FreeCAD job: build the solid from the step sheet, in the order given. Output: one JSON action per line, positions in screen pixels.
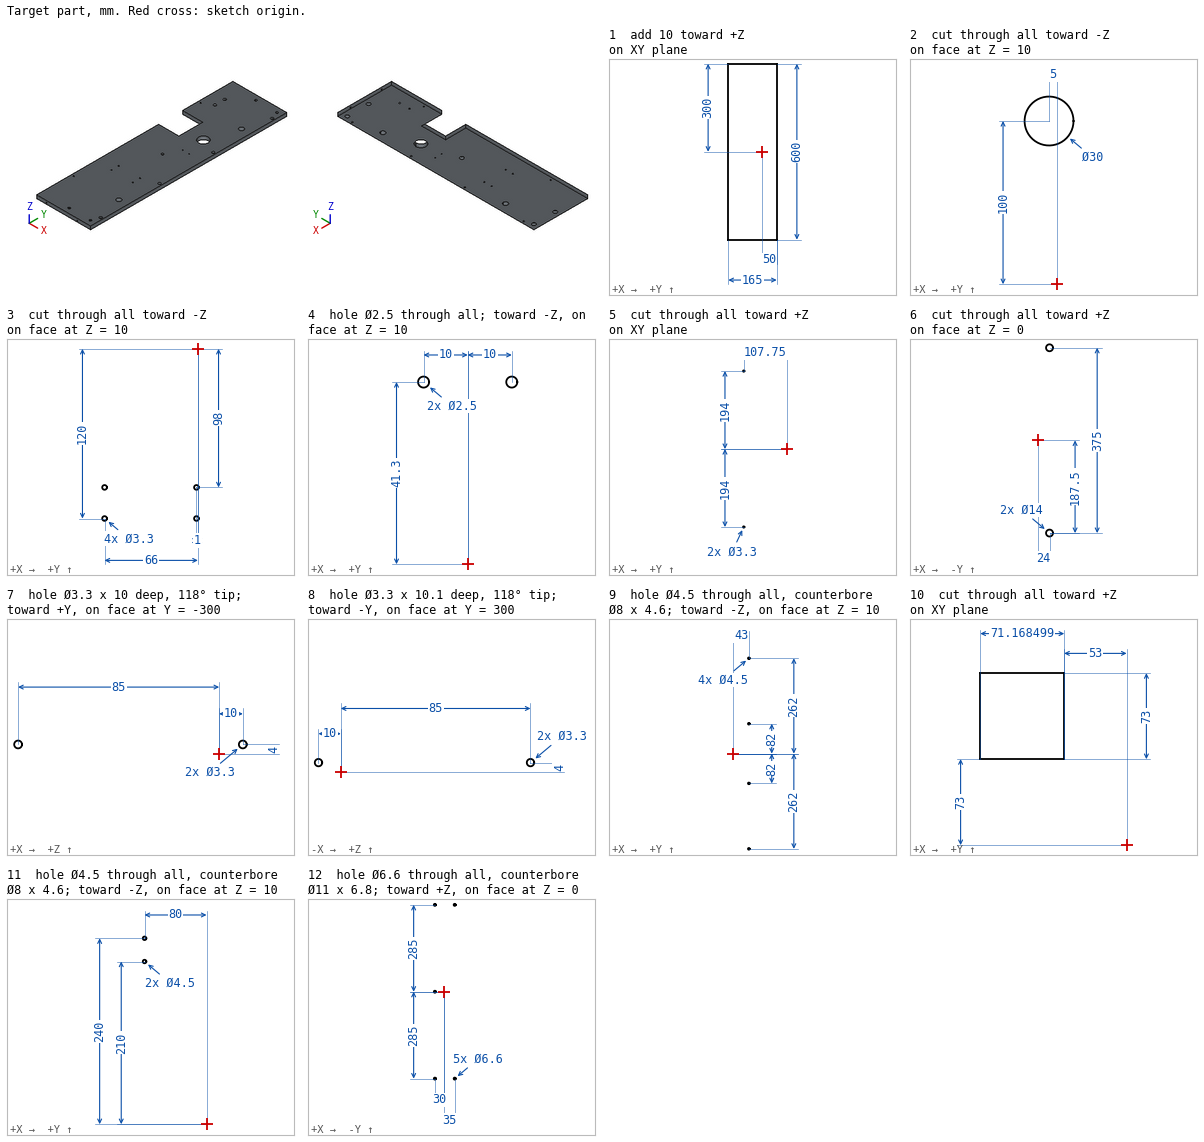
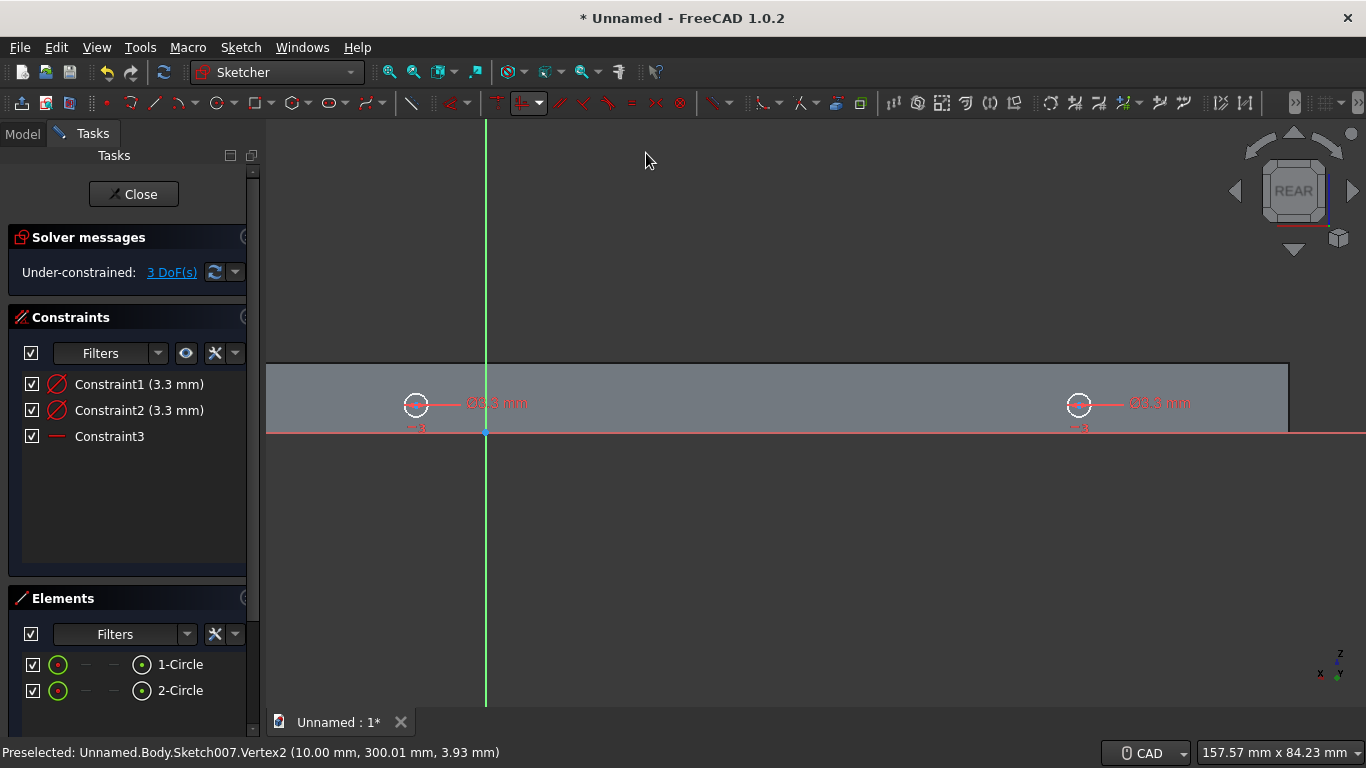
{"action": "left_click", "coordinate": [450, 104]}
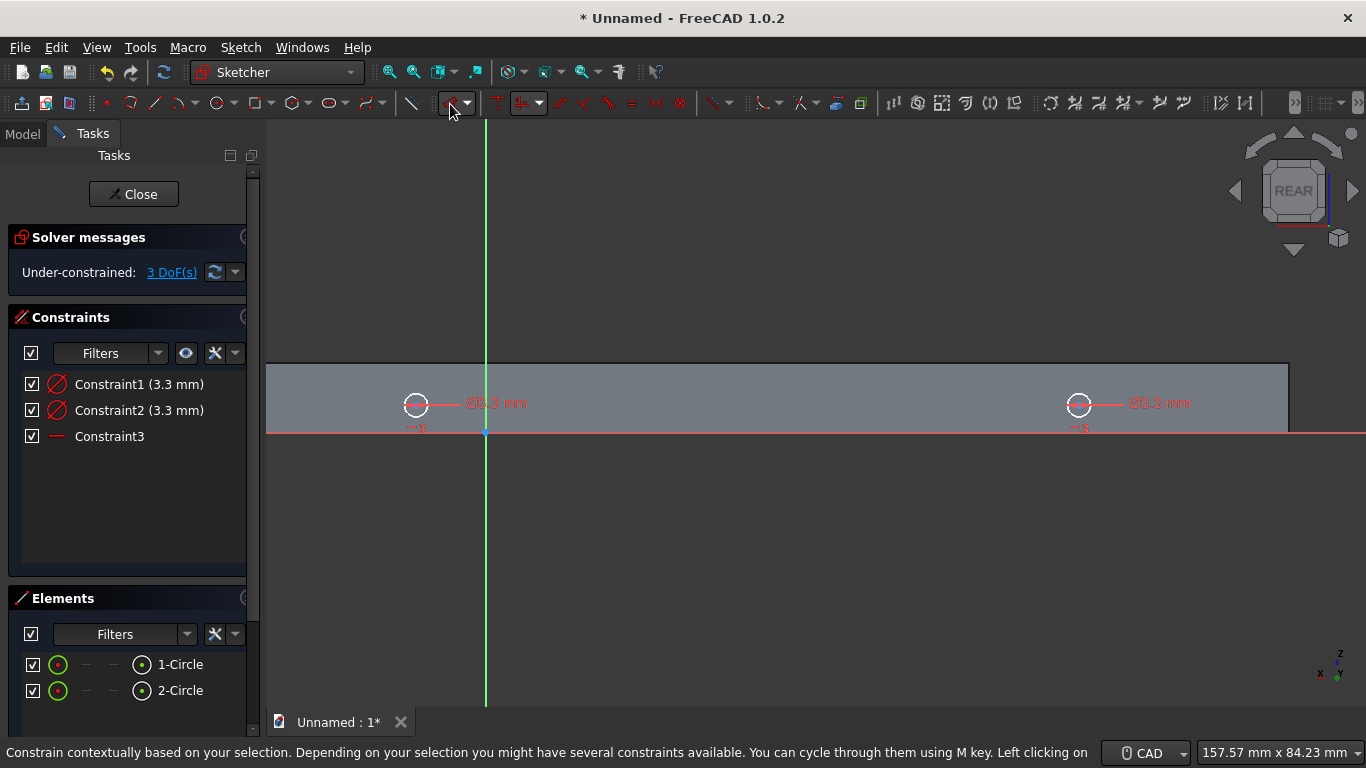
{"action": "scroll", "coordinate": [1079, 405], "scroll_direction": "up", "scroll_amount": 2}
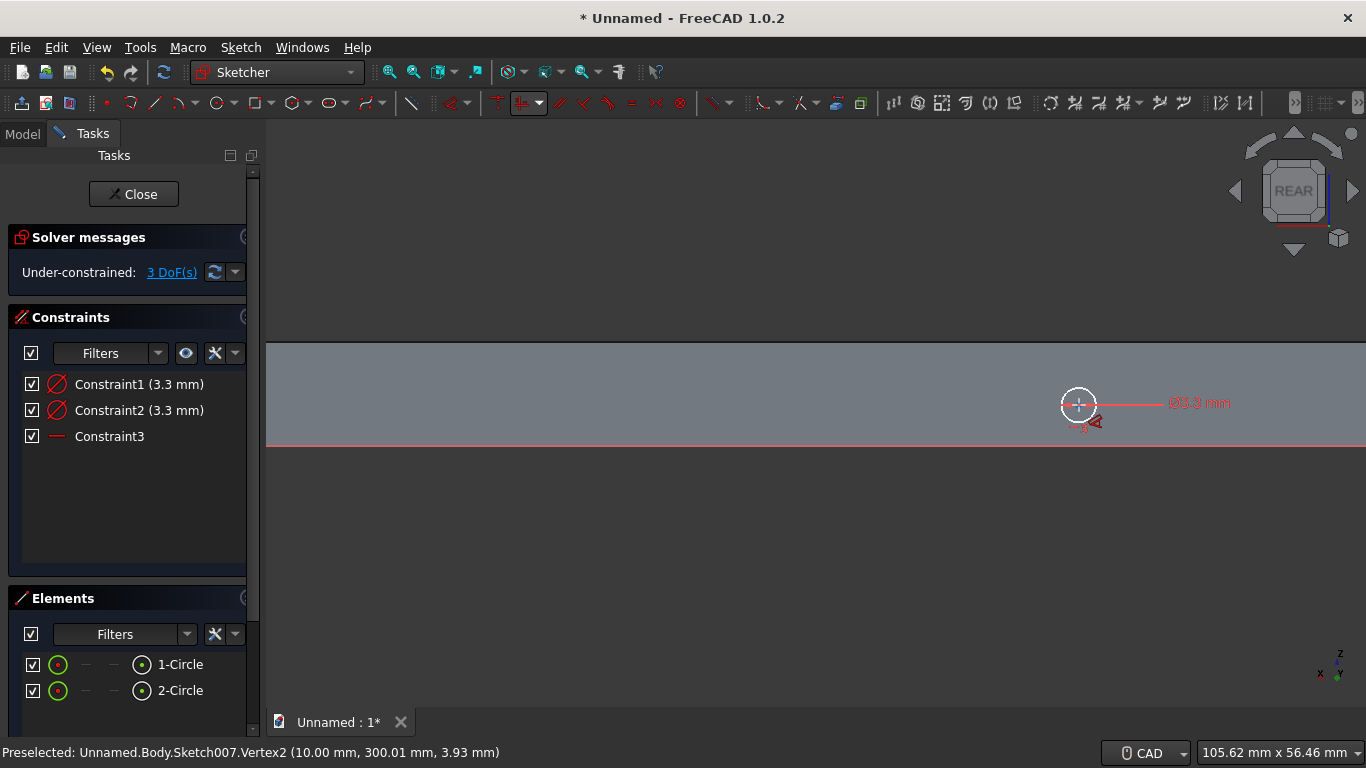
{"action": "left_click", "coordinate": [1079, 405]}
{"action": "left_click", "coordinate": [1113, 426]}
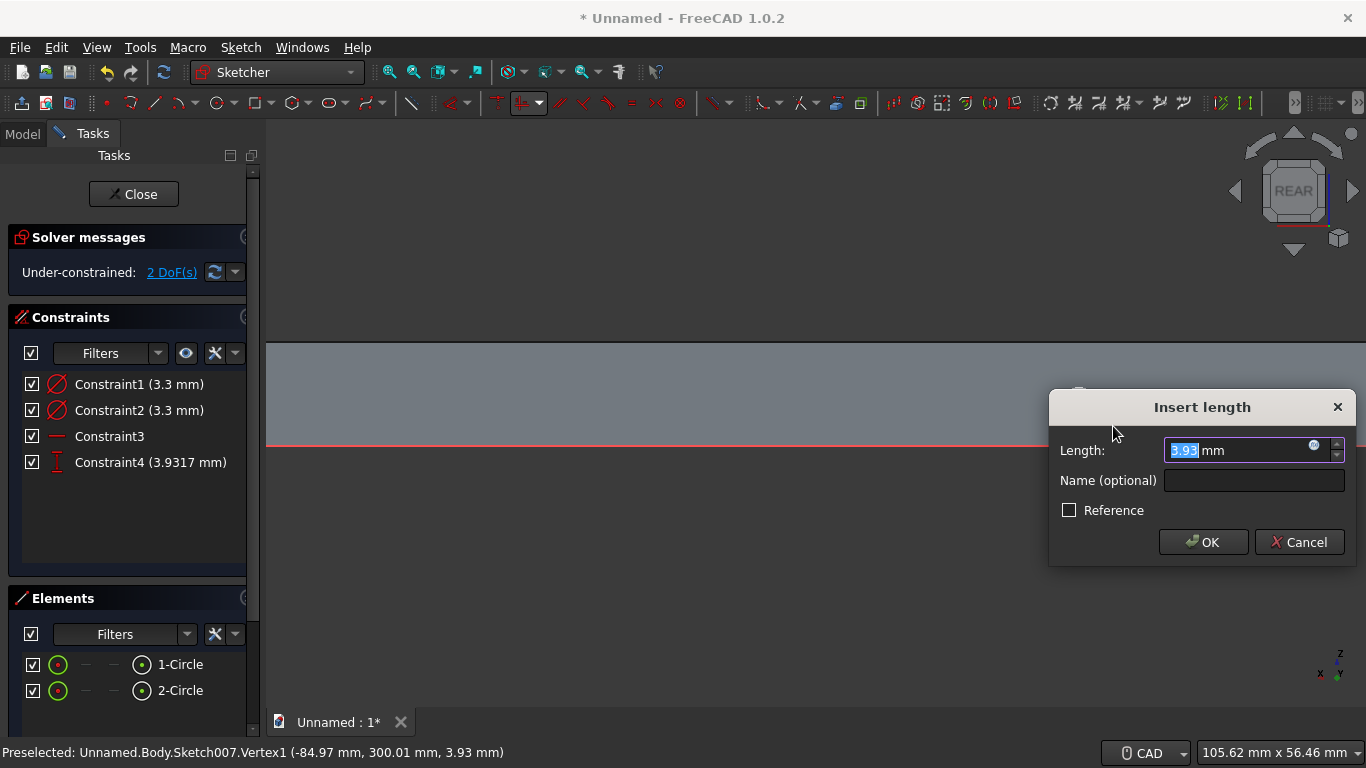
{"action": "type", "text": "4"}
{"action": "key", "text": "Return"}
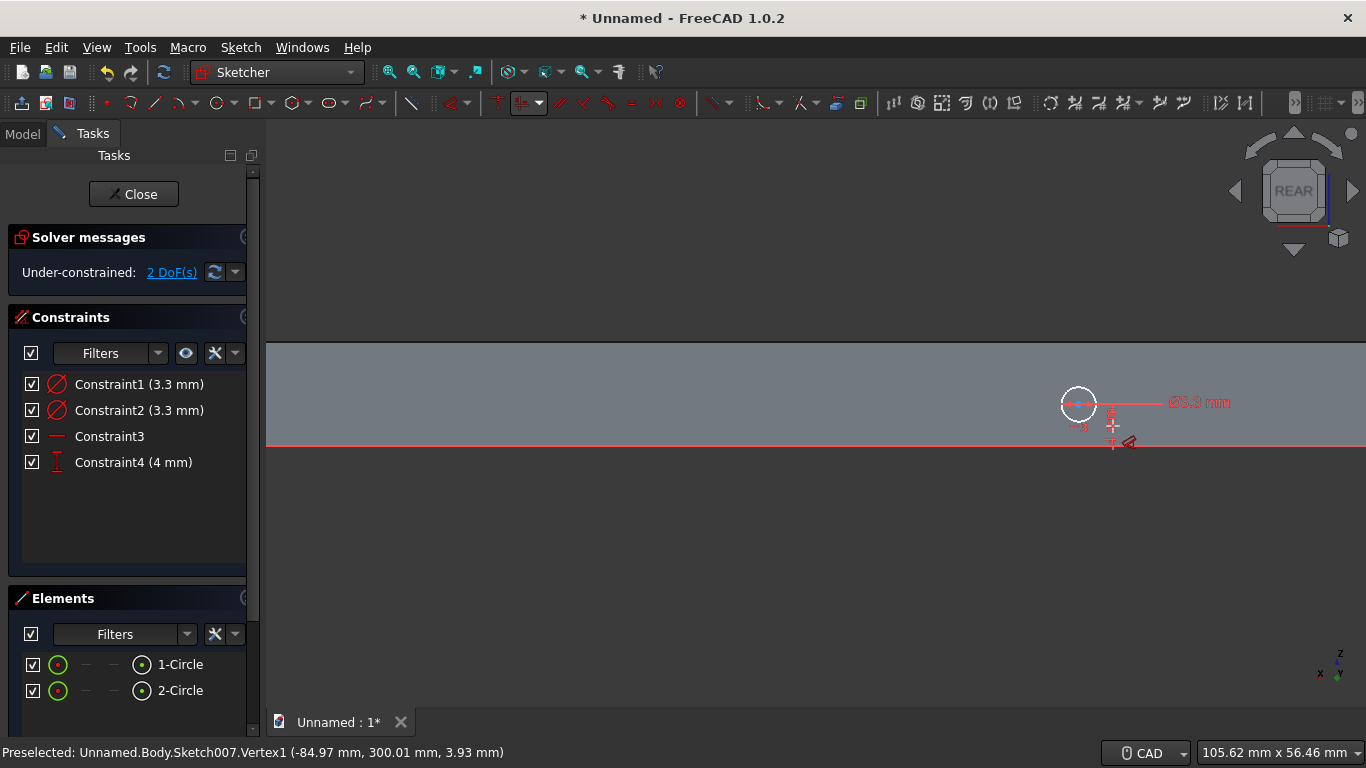
{"action": "left_click", "coordinate": [1079, 404]}
{"action": "left_click", "coordinate": [686, 480]}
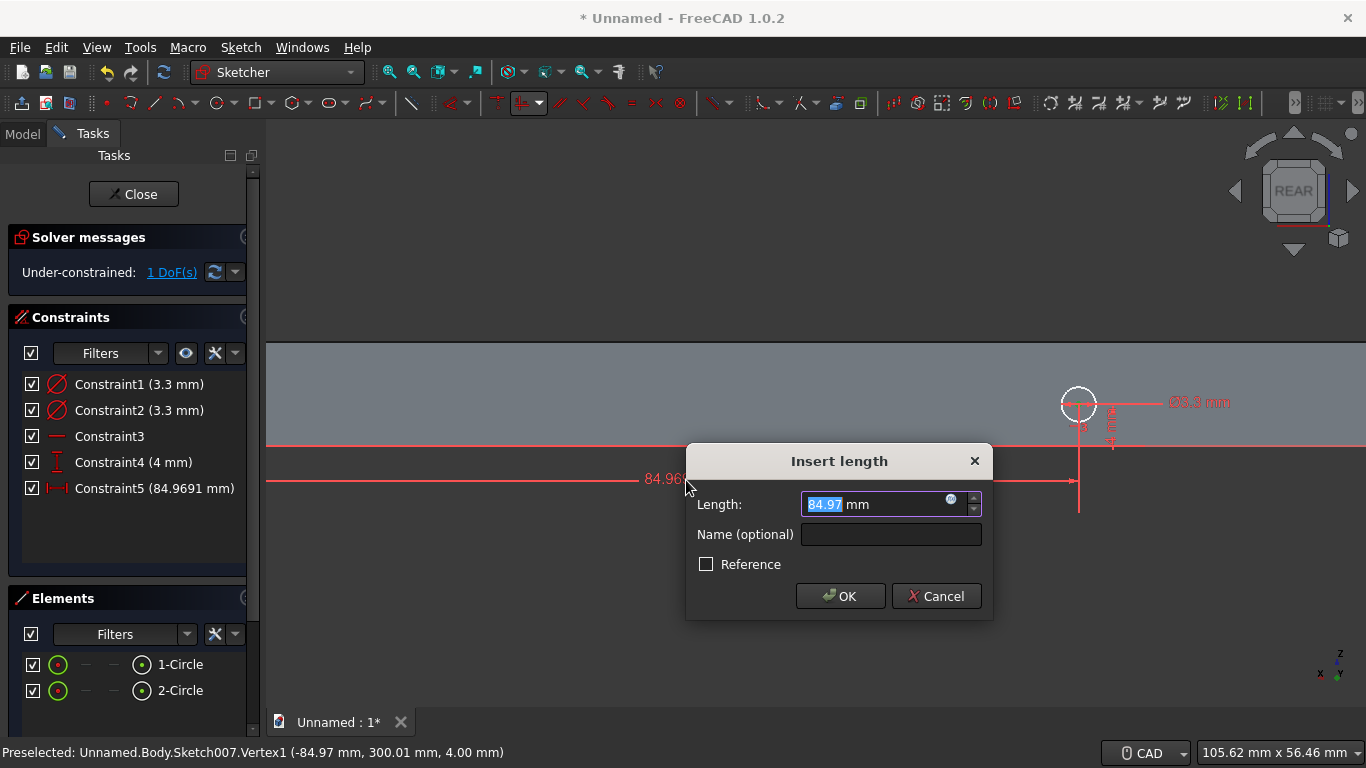
{"action": "type", "text": "85"}
{"action": "key", "text": "Return"}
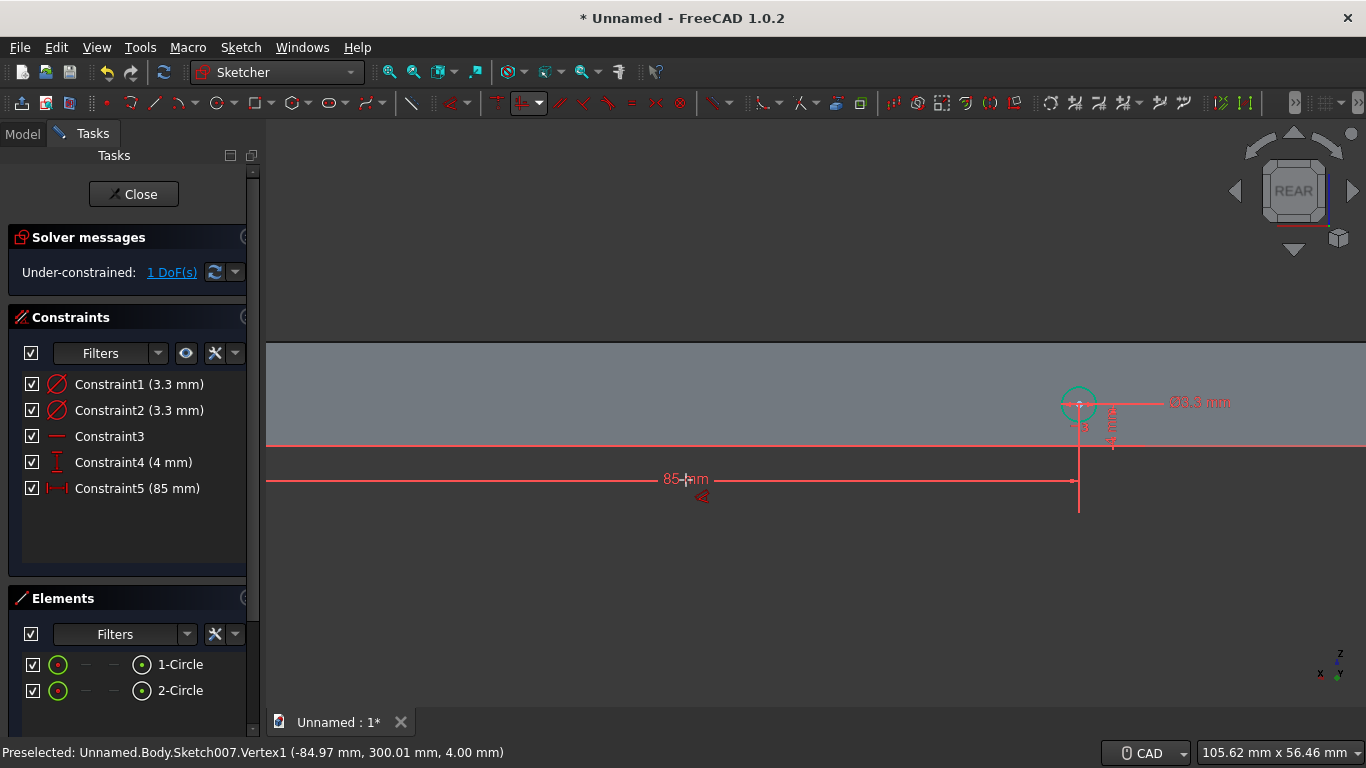
{"action": "scroll", "coordinate": [1079, 406], "scroll_direction": "down", "scroll_amount": 2}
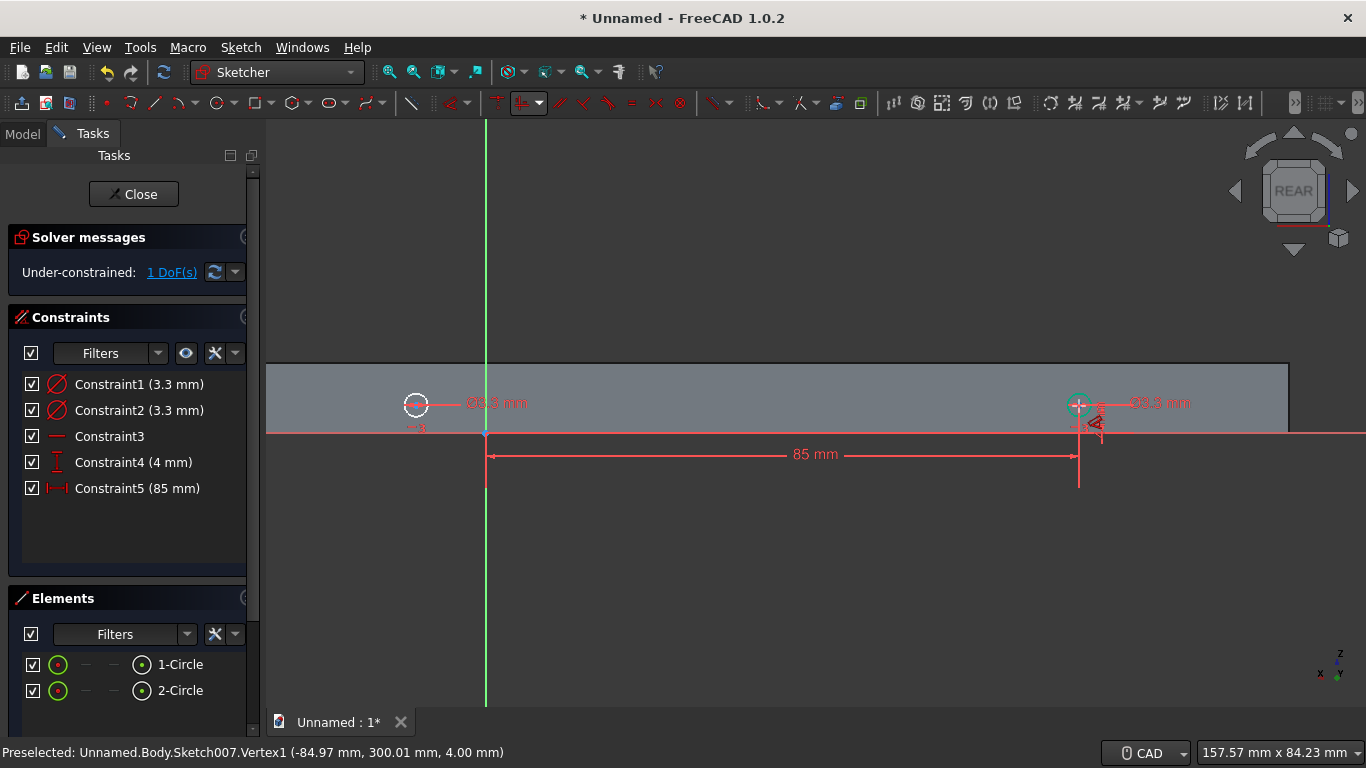
{"action": "left_click", "coordinate": [416, 405]}
{"action": "left_click", "coordinate": [451, 467]}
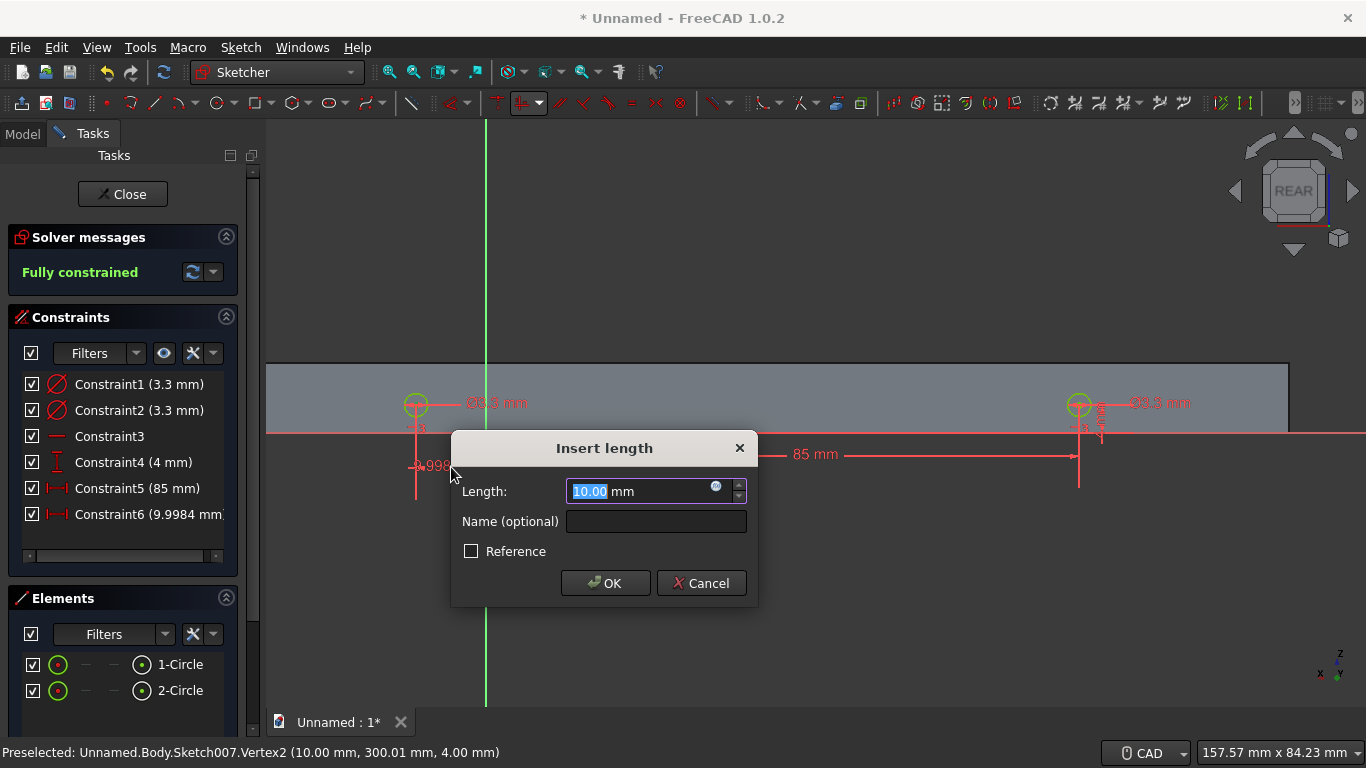
{"action": "type", "text": "10"}
{"action": "key", "text": "Return"}
{"action": "key", "text": "Escape"}